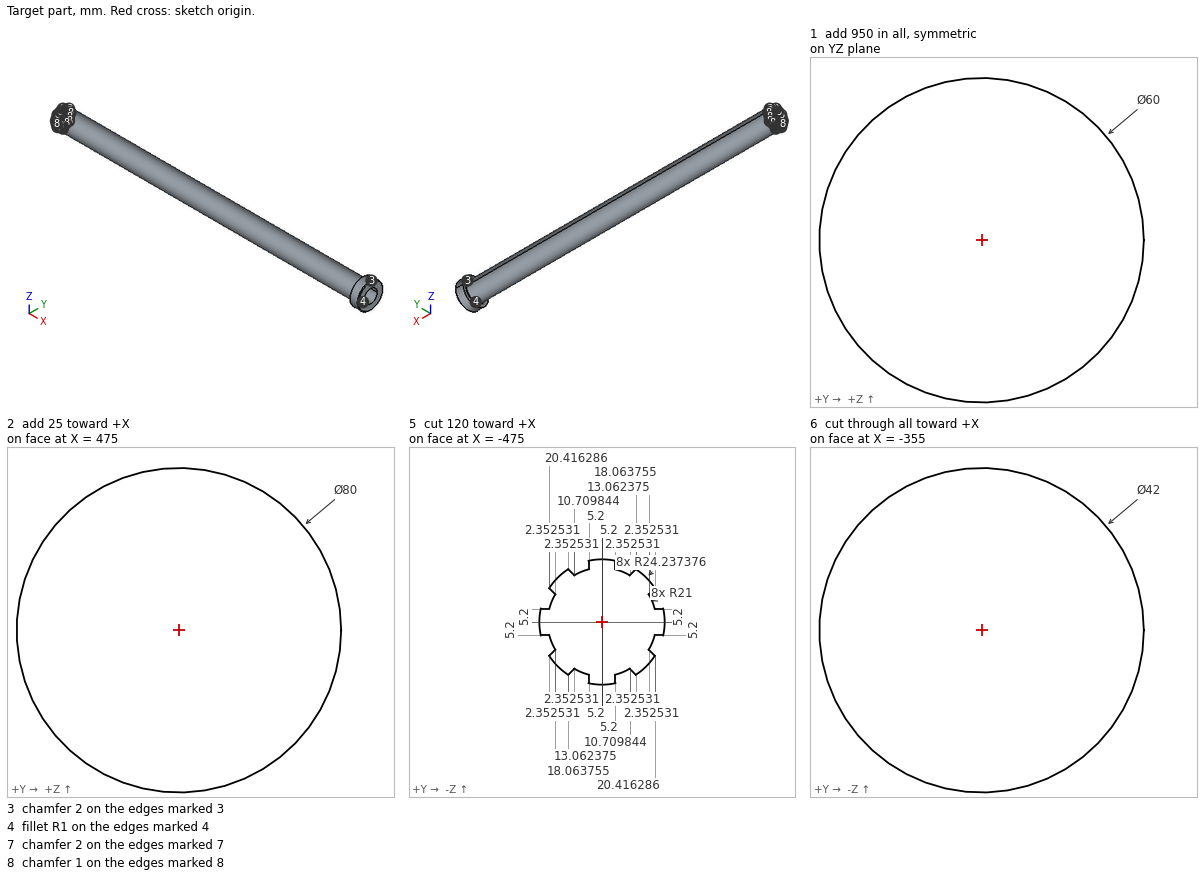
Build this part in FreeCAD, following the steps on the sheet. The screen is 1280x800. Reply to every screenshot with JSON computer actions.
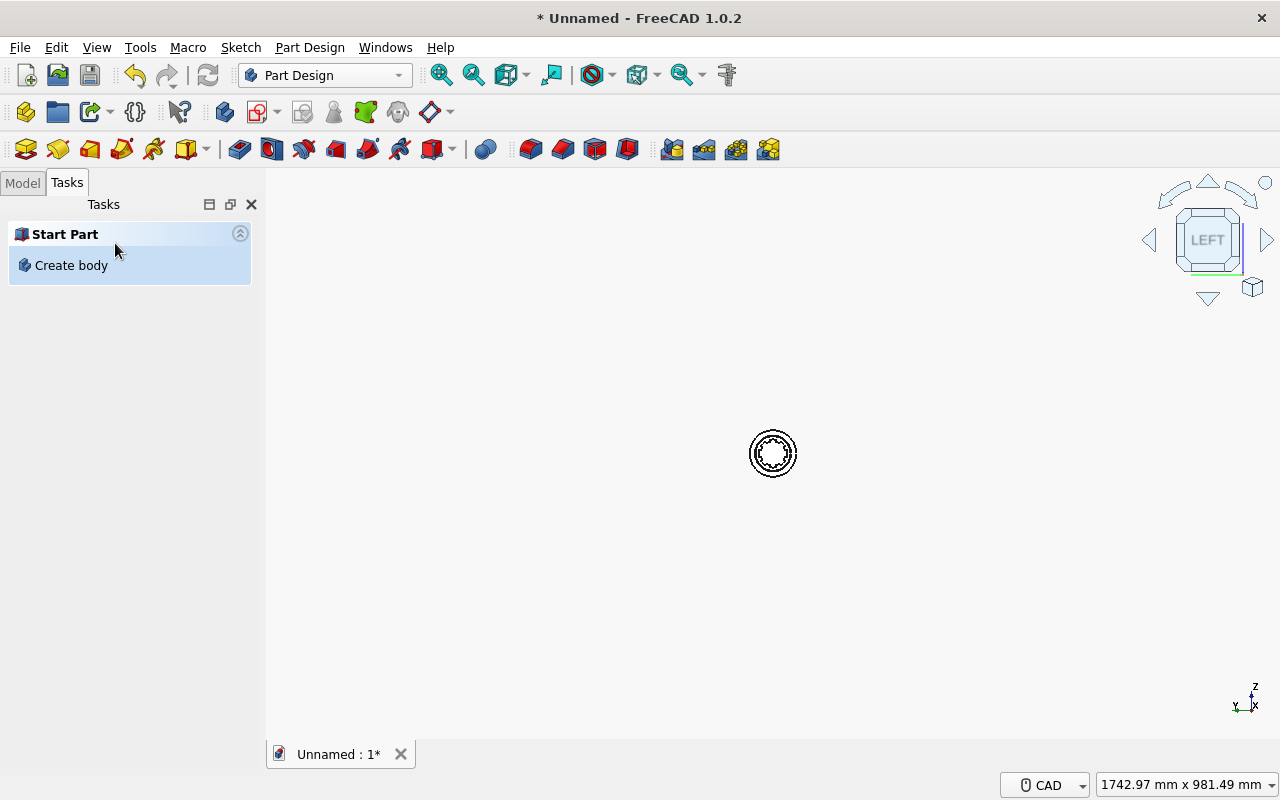
{"action": "left_click", "coordinate": [442, 76]}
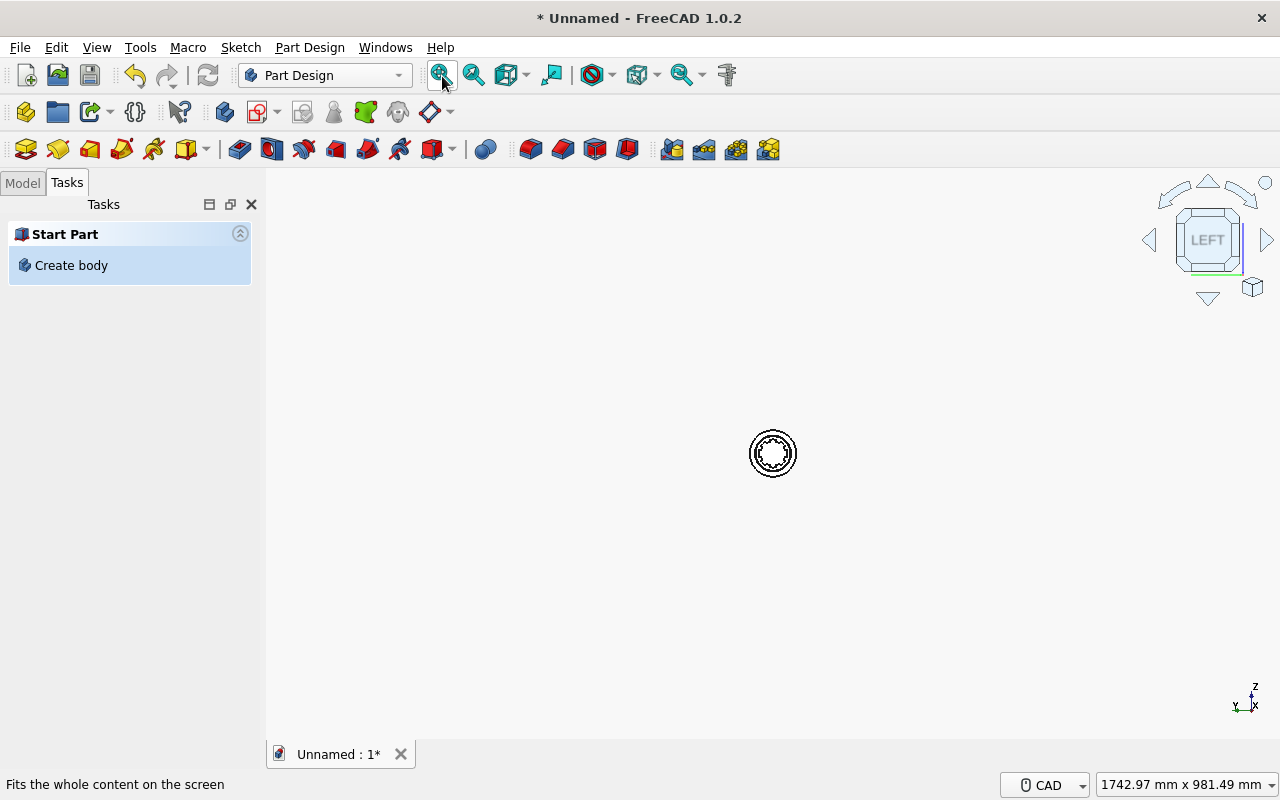
{"action": "left_click", "coordinate": [773, 452]}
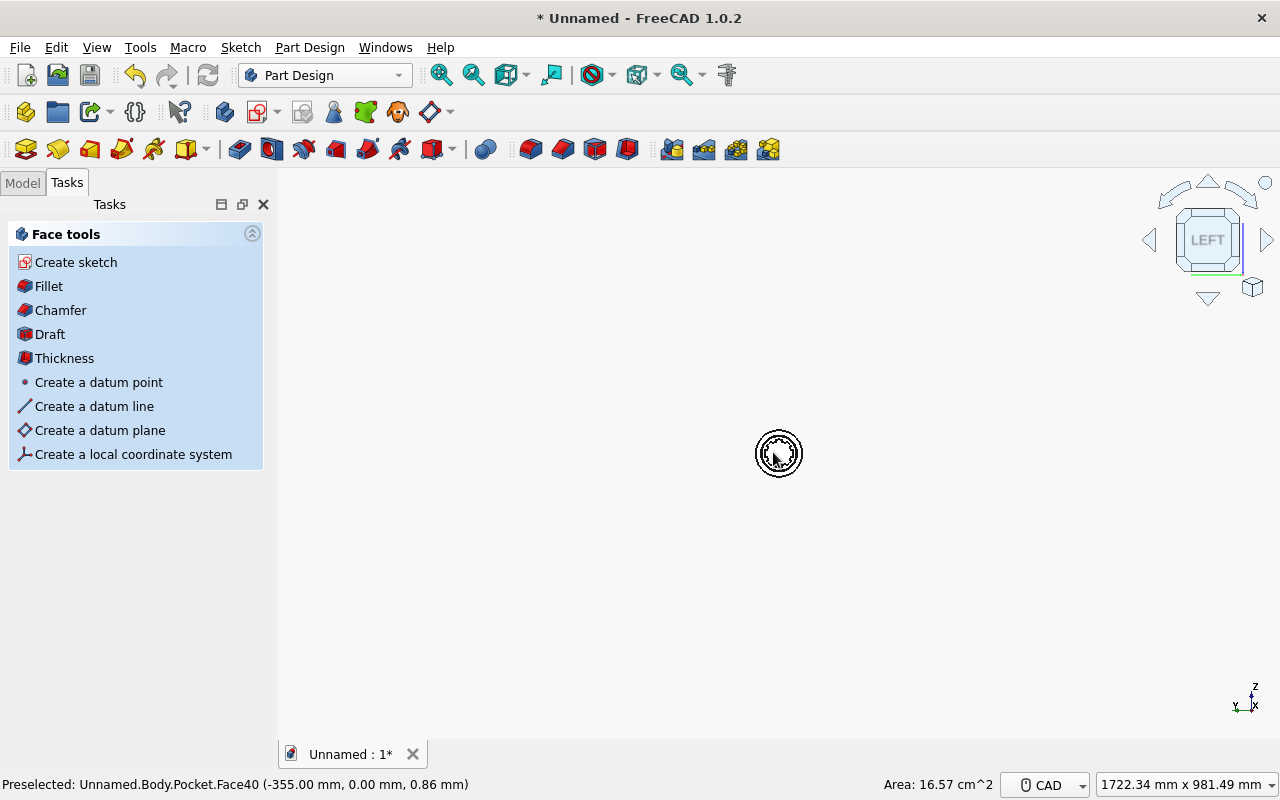
{"action": "left_click", "coordinate": [258, 112]}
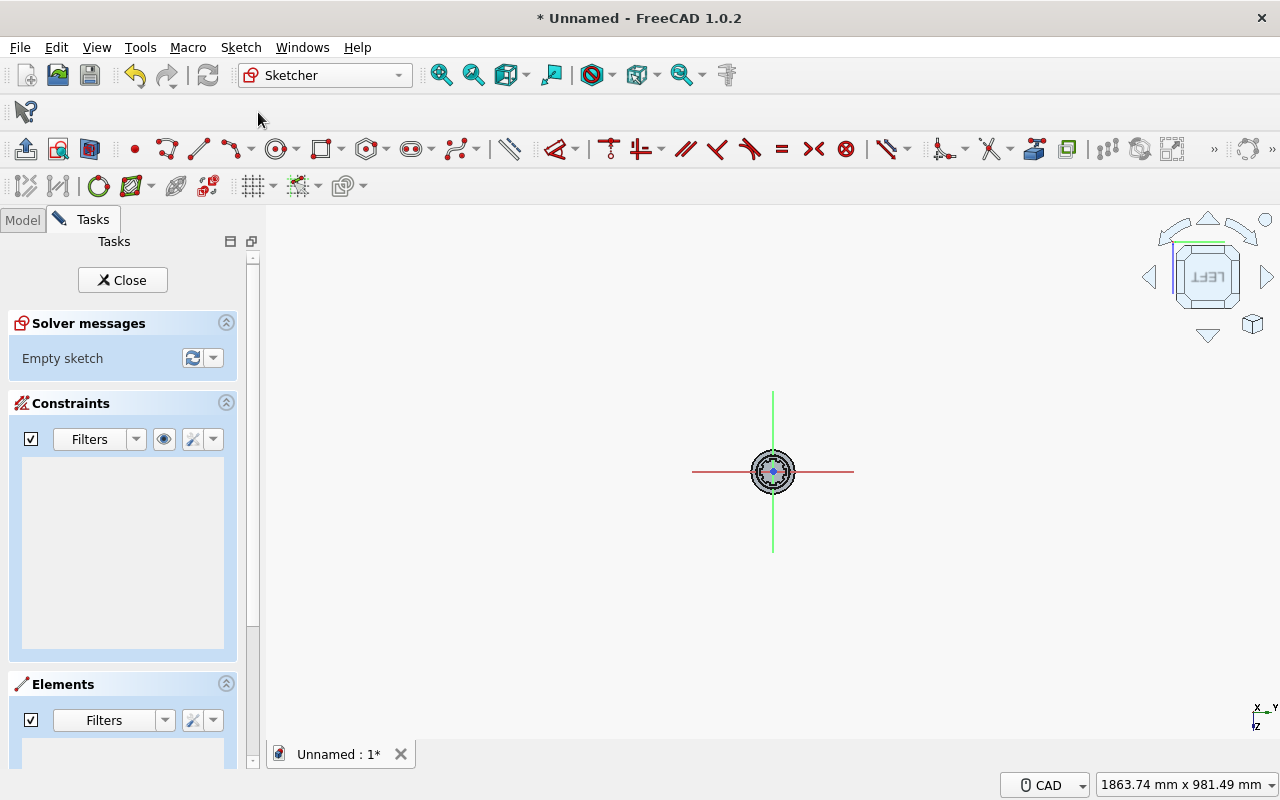
{"action": "left_click", "coordinate": [90, 150]}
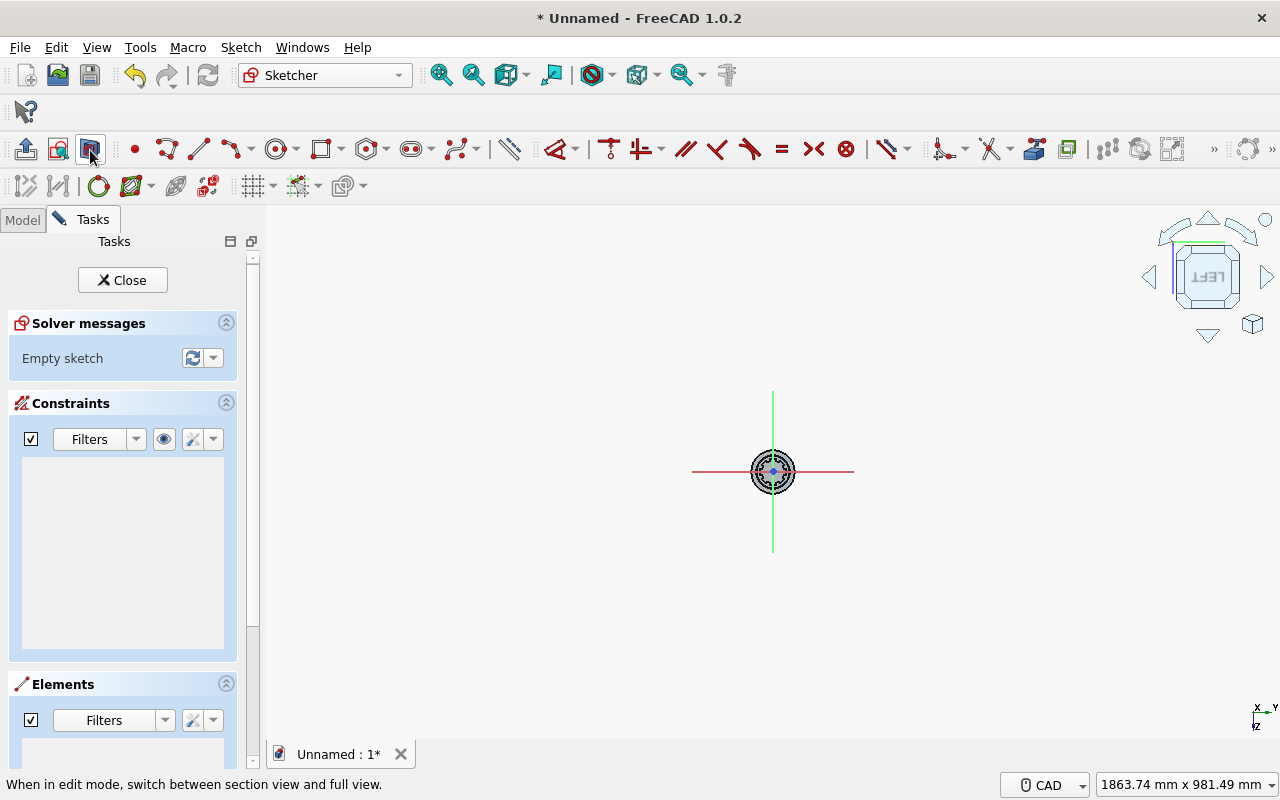
{"action": "scroll", "coordinate": [778, 472], "scroll_direction": "up", "scroll_amount": 13}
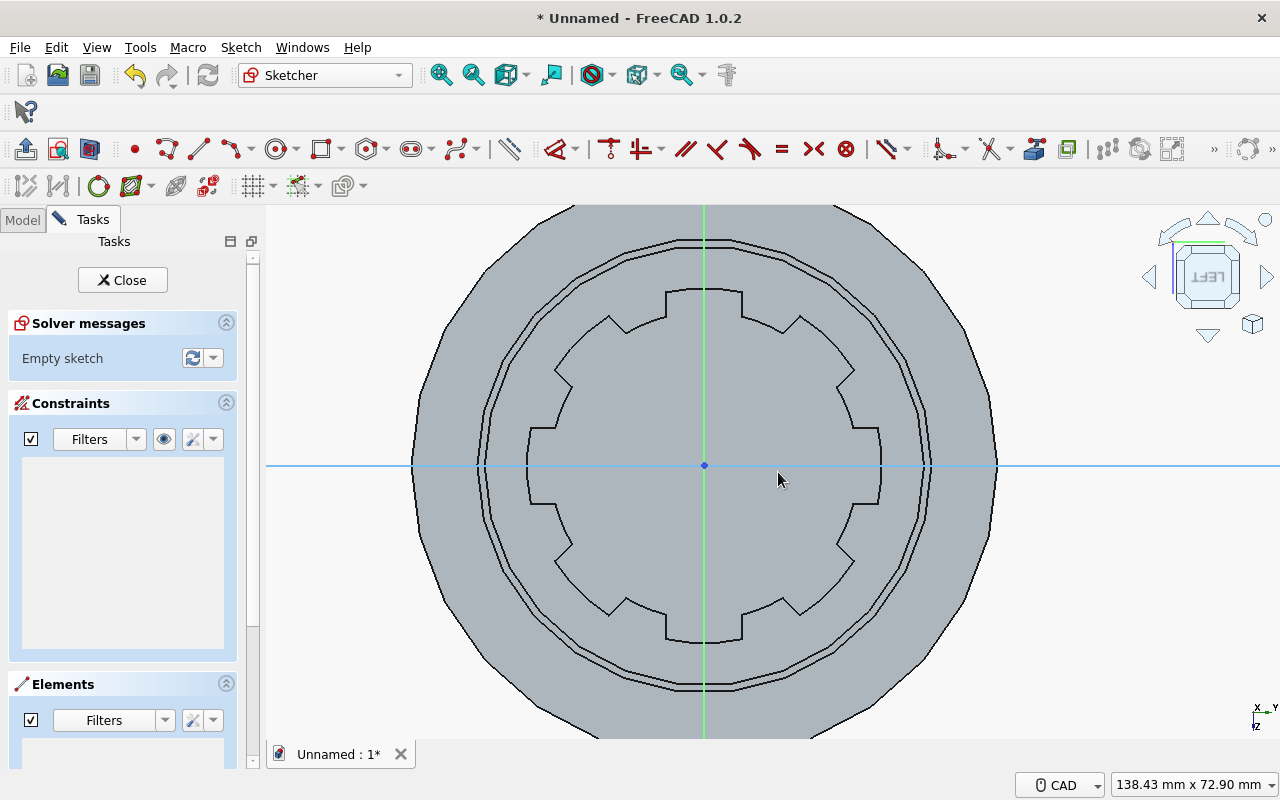
{"action": "key", "text": "g c"}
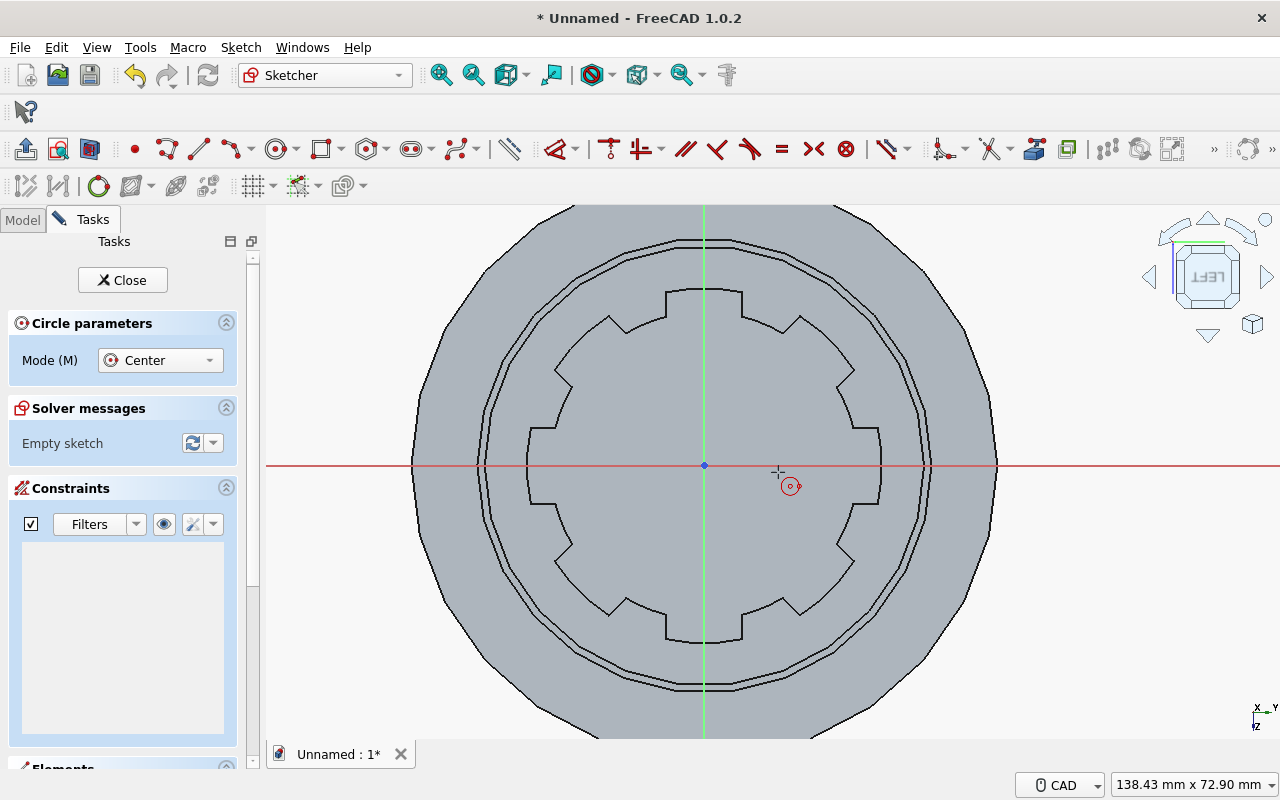
{"action": "left_click", "coordinate": [704, 466]}
{"action": "mouse_move", "coordinate": [813, 357]}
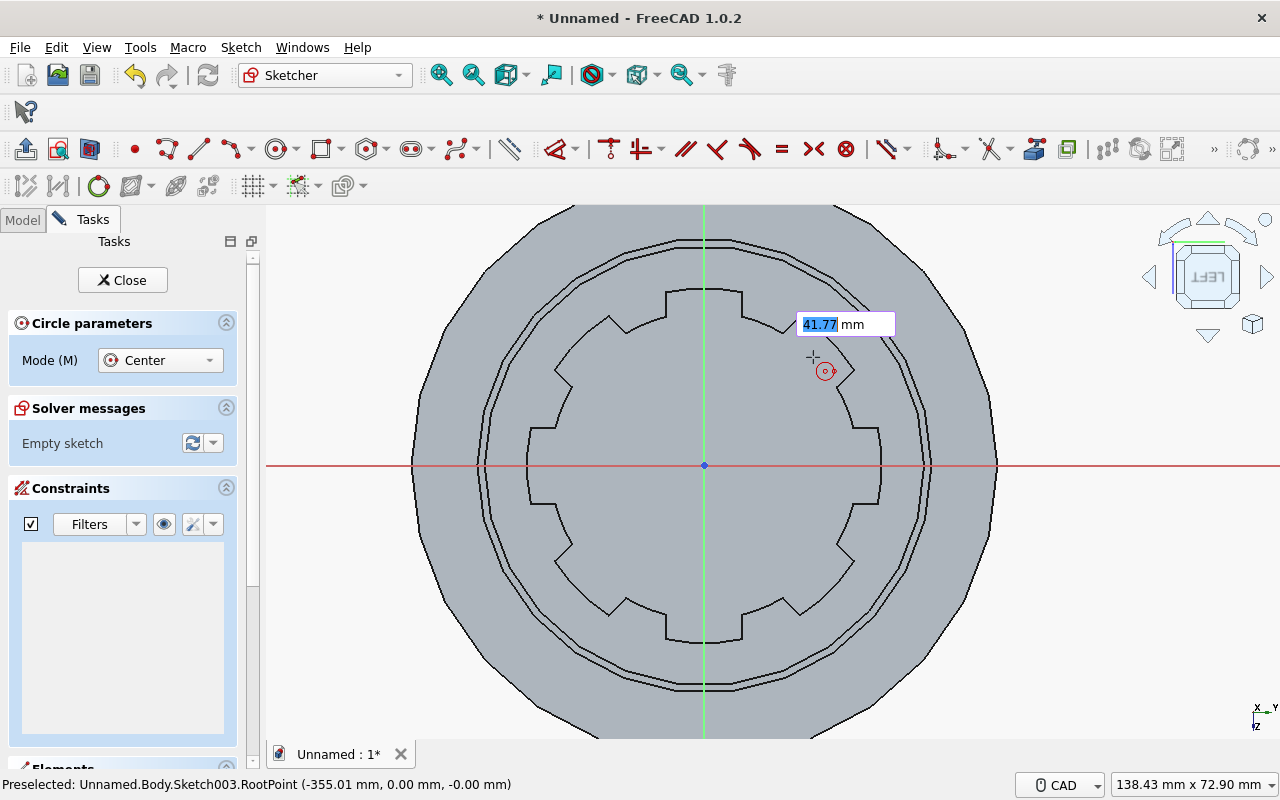
{"action": "type", "text": "42"}
{"action": "key", "text": "Return"}
{"action": "key", "text": "Escape"}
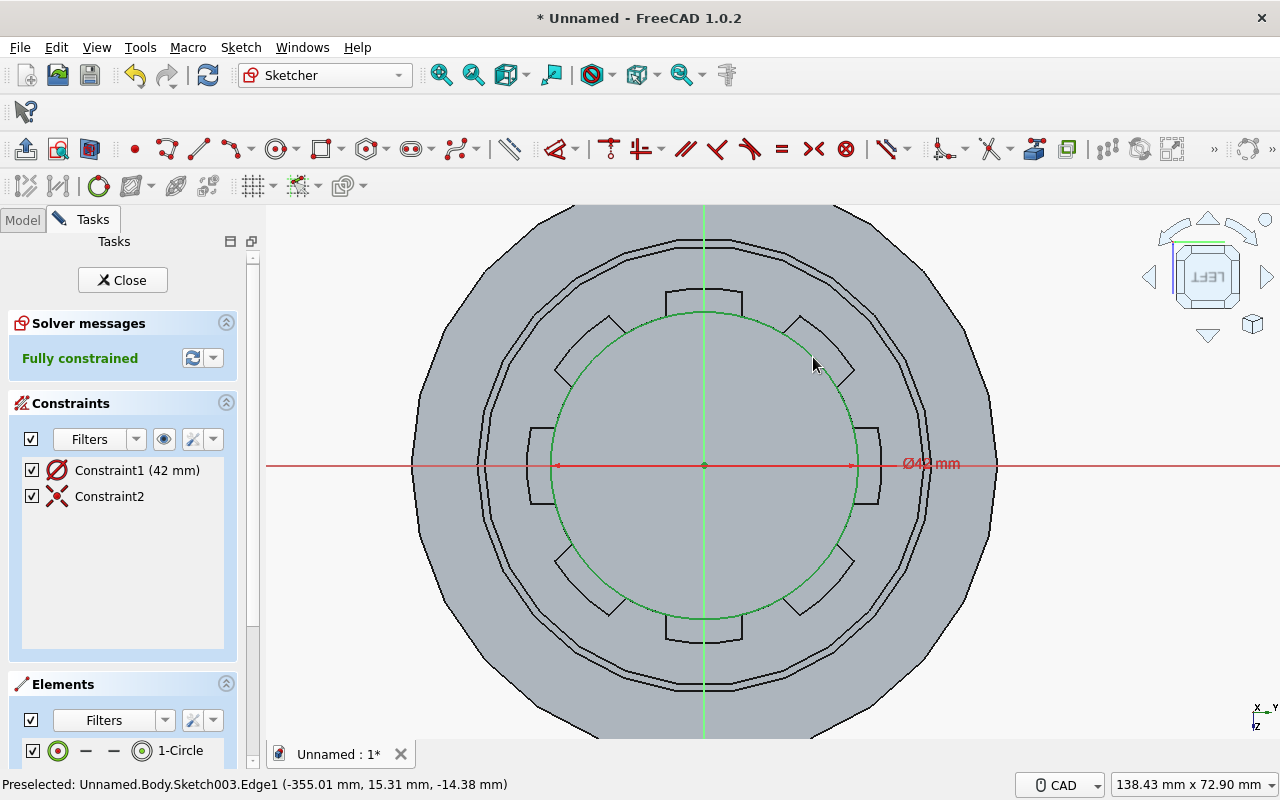
{"action": "left_click", "coordinate": [123, 280]}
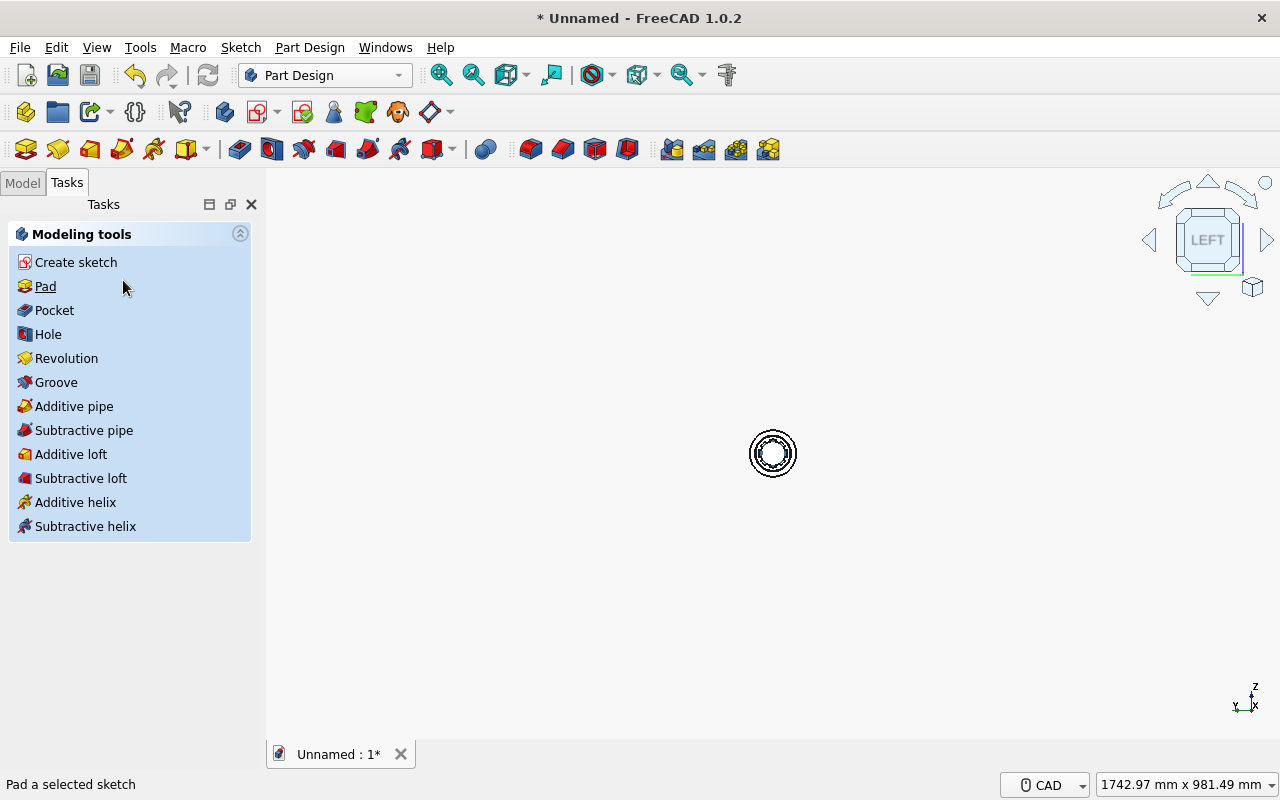
{"action": "left_click", "coordinate": [240, 150]}